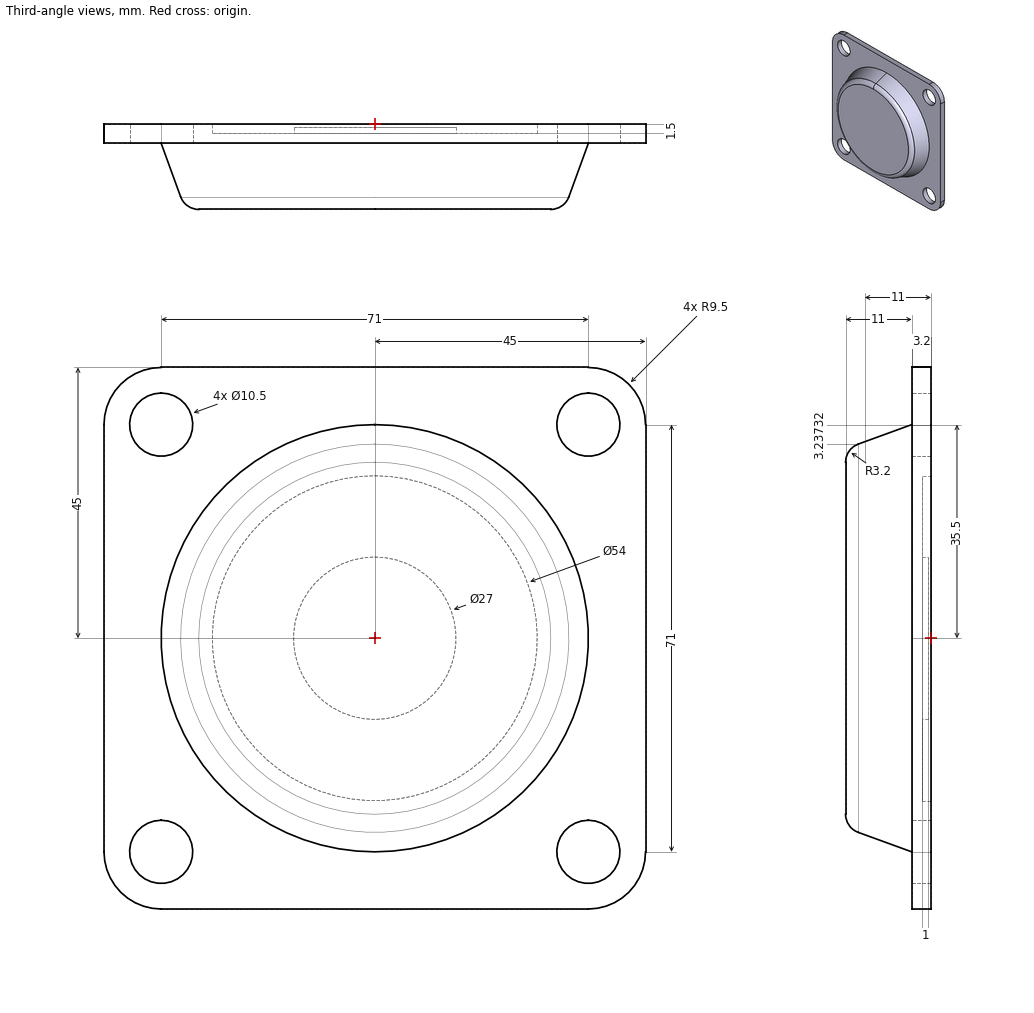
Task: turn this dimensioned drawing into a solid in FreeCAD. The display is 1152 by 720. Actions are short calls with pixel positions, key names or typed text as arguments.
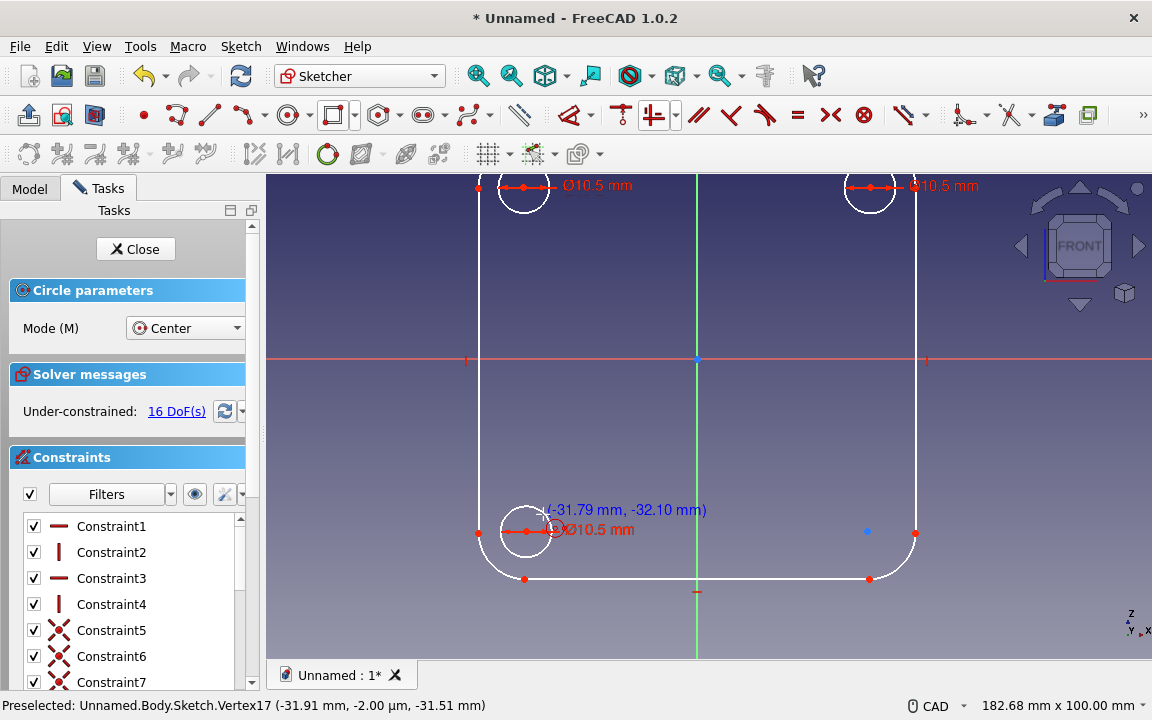
click(869, 532)
move(887, 514)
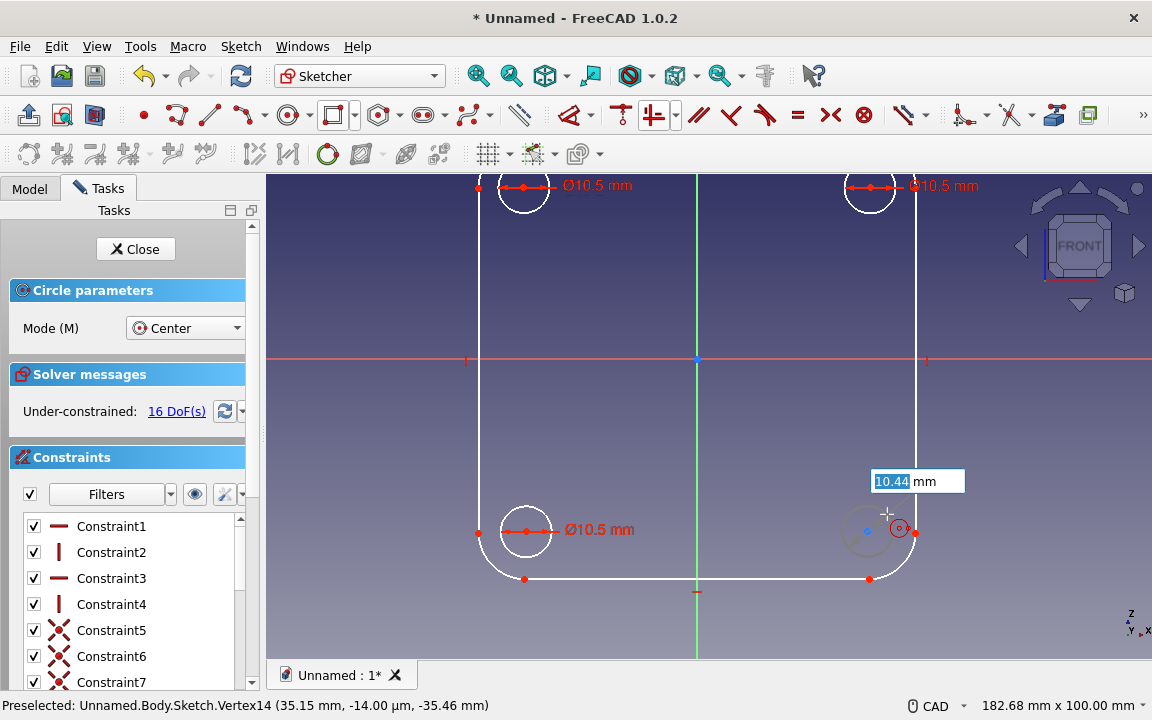
text(10.5)
key(Return)
key(Escape)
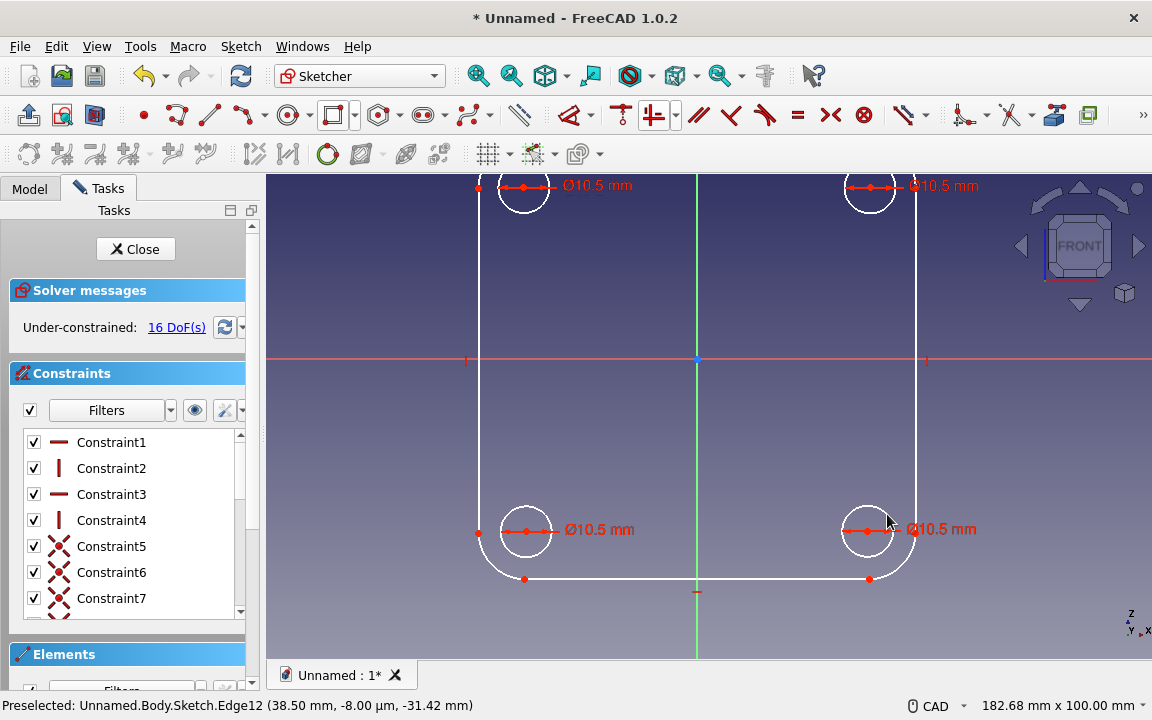
scroll(525, 533, down, 2)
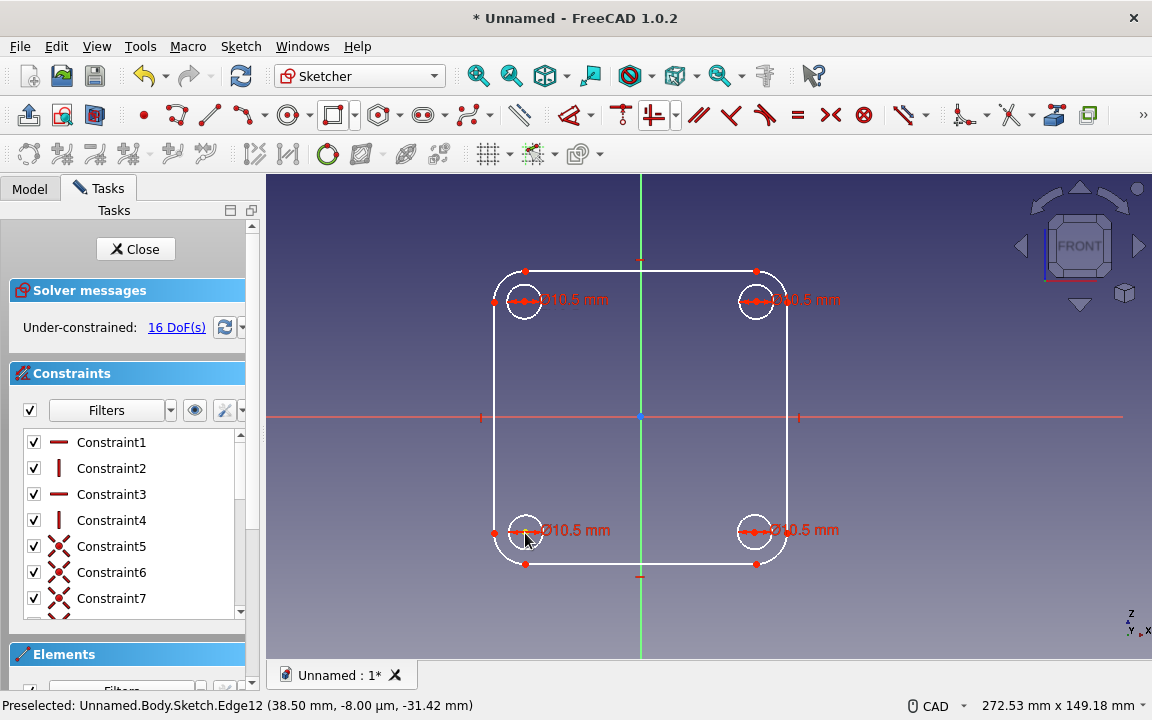
click(594, 271)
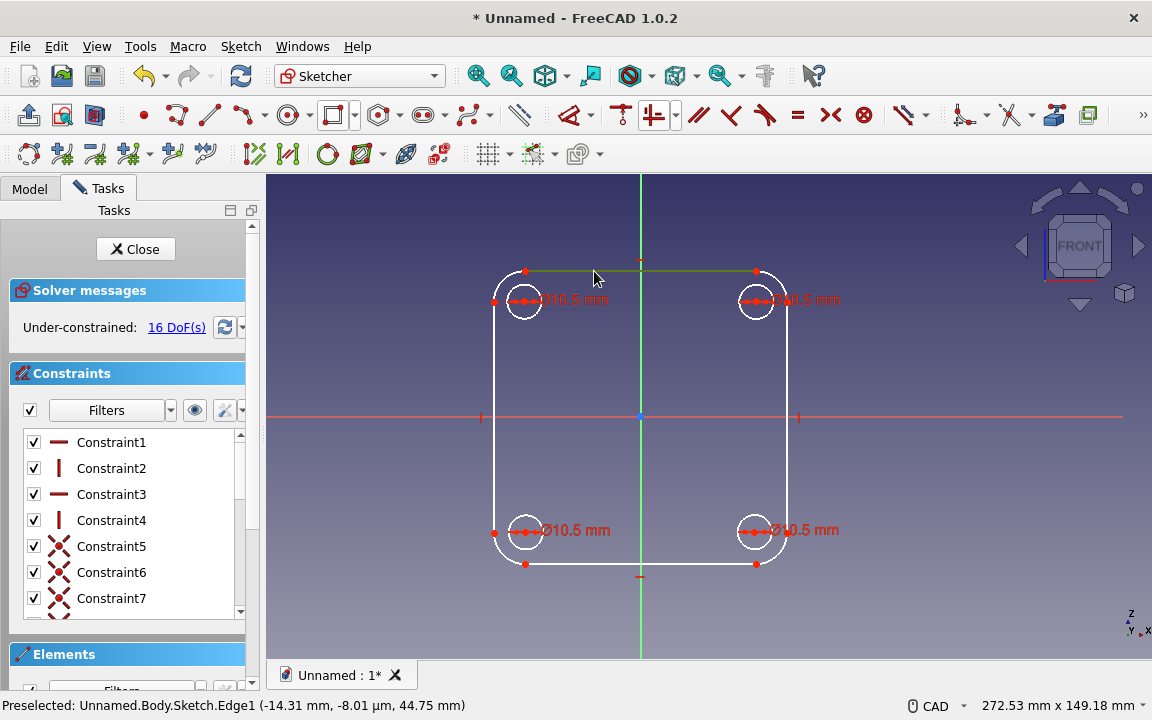
click(784, 288)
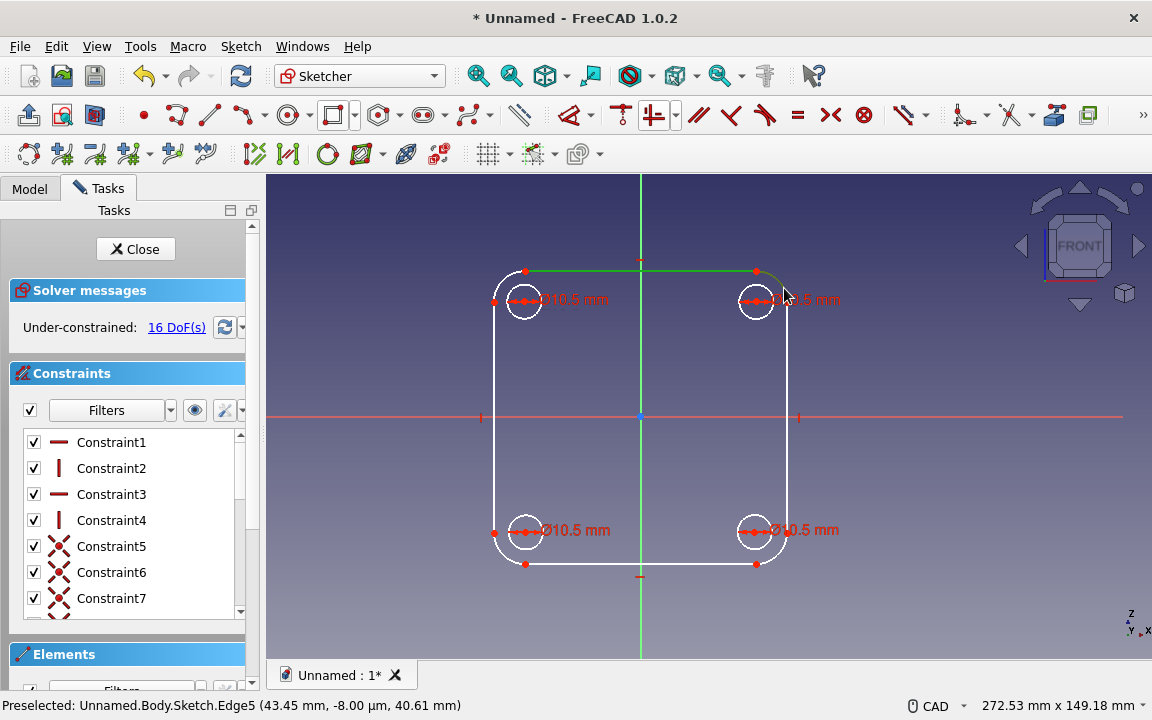
key(t)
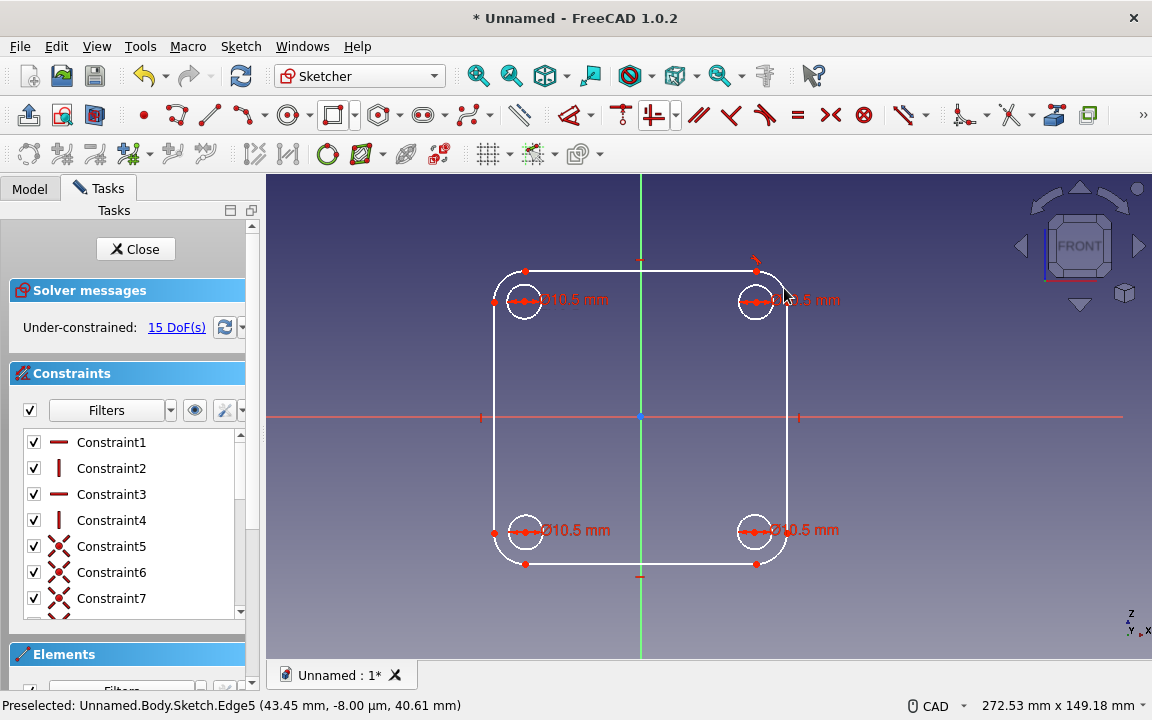
click(594, 271)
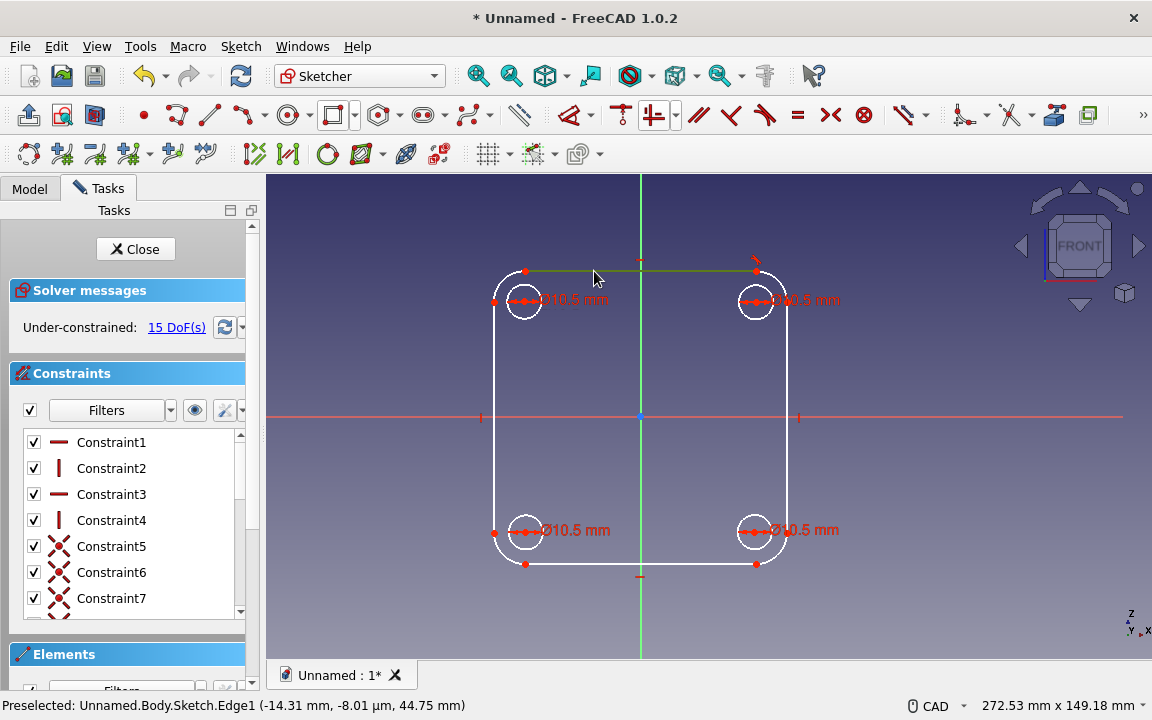
click(511, 275)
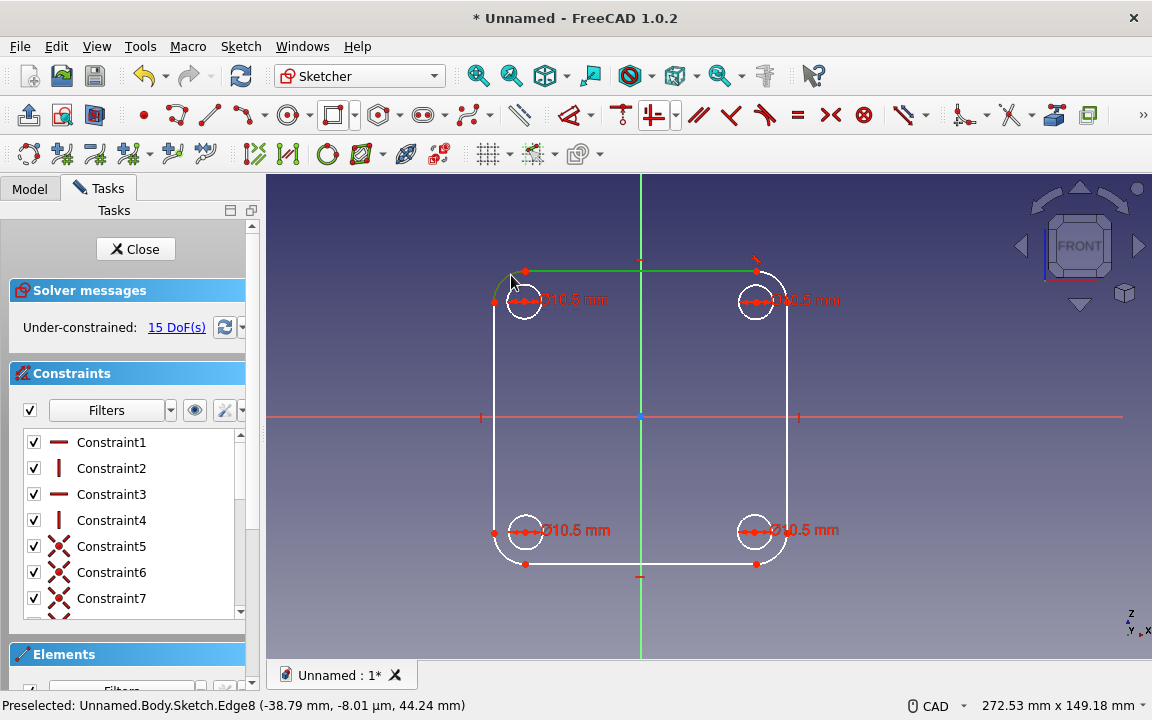
click(765, 116)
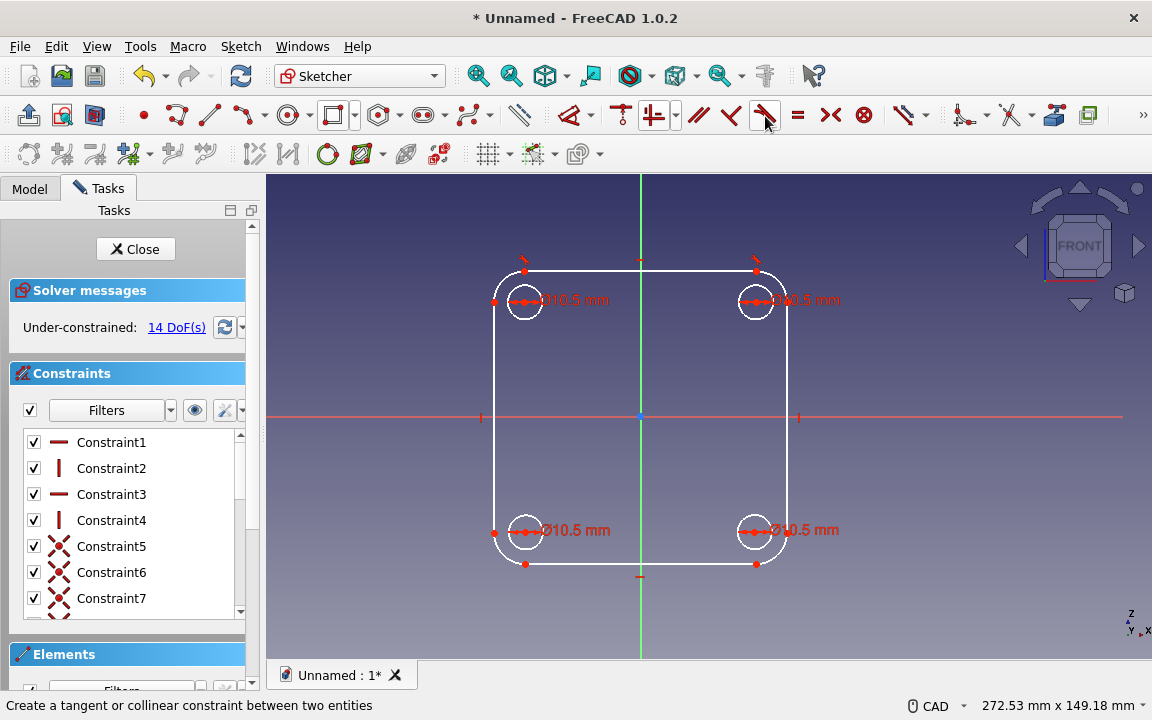
click(787, 372)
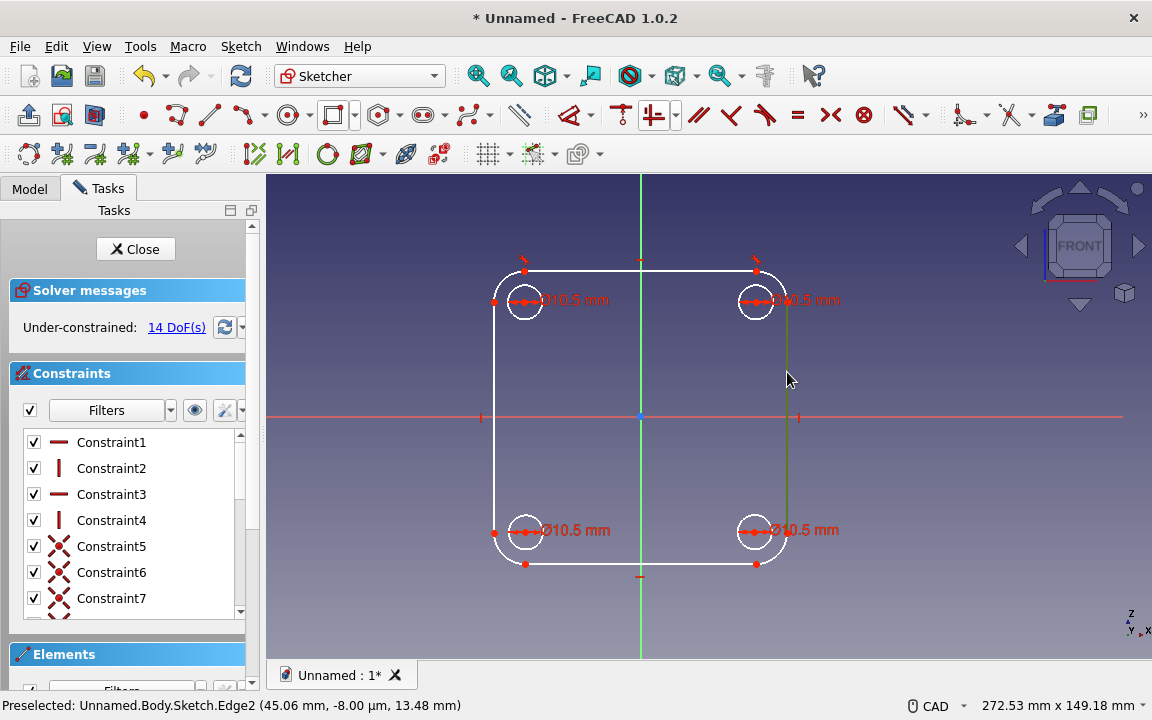
click(784, 288)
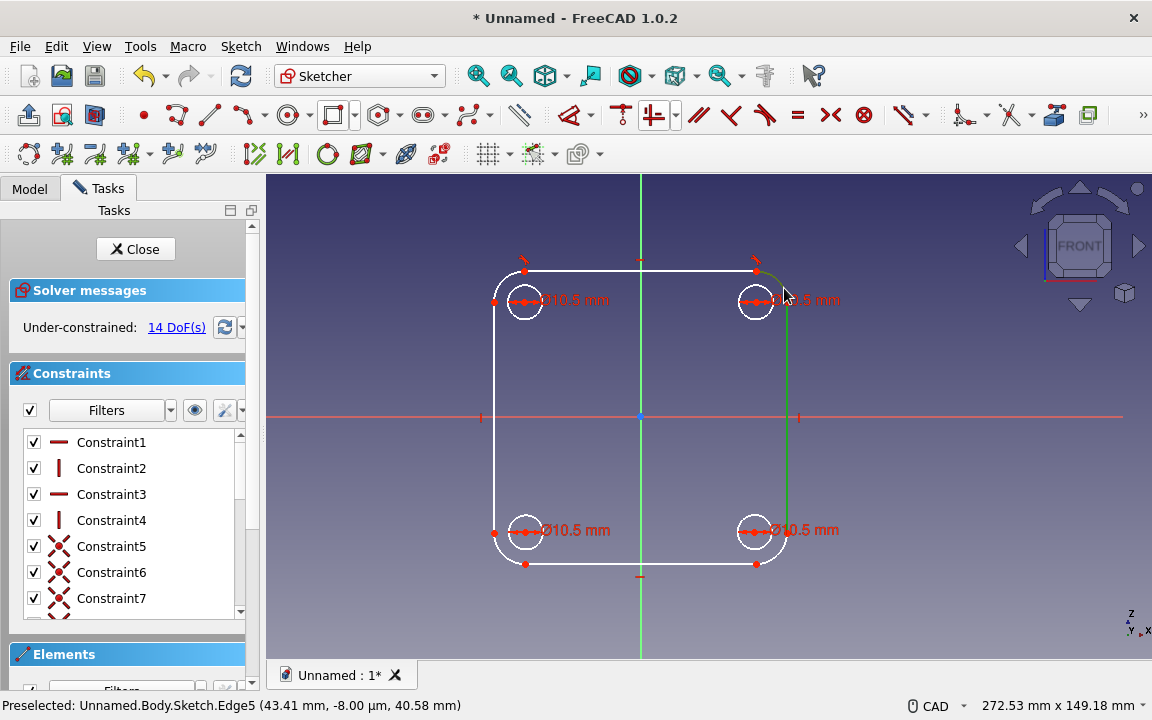
key(t)